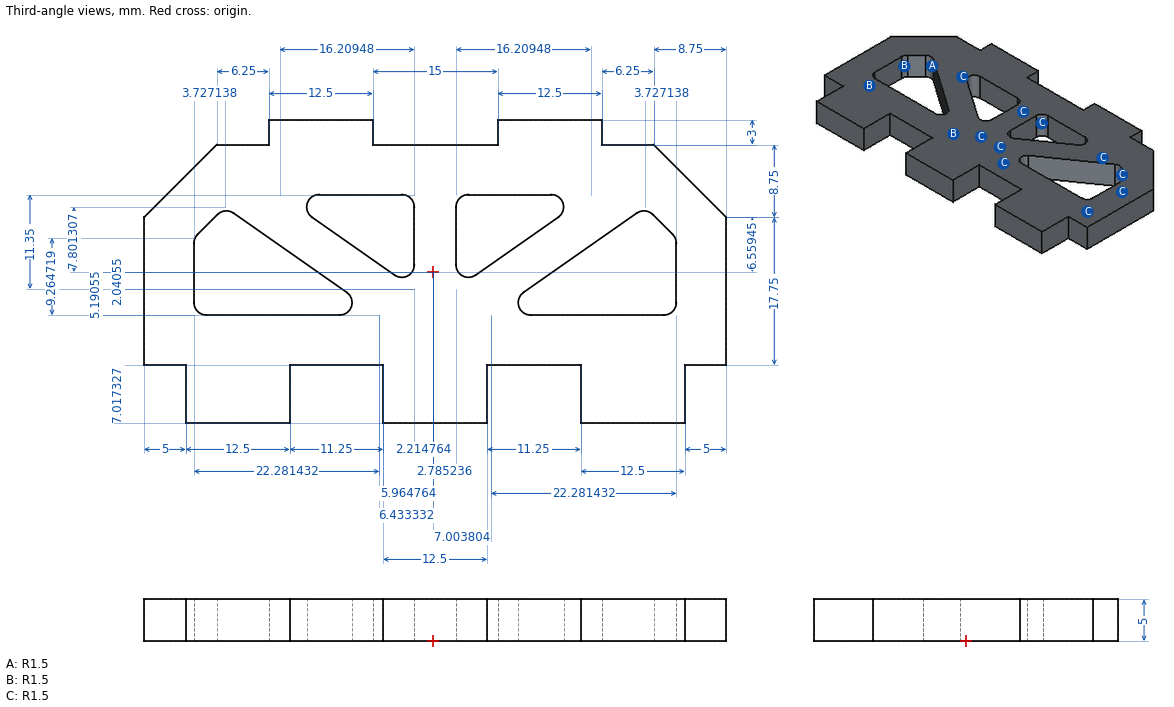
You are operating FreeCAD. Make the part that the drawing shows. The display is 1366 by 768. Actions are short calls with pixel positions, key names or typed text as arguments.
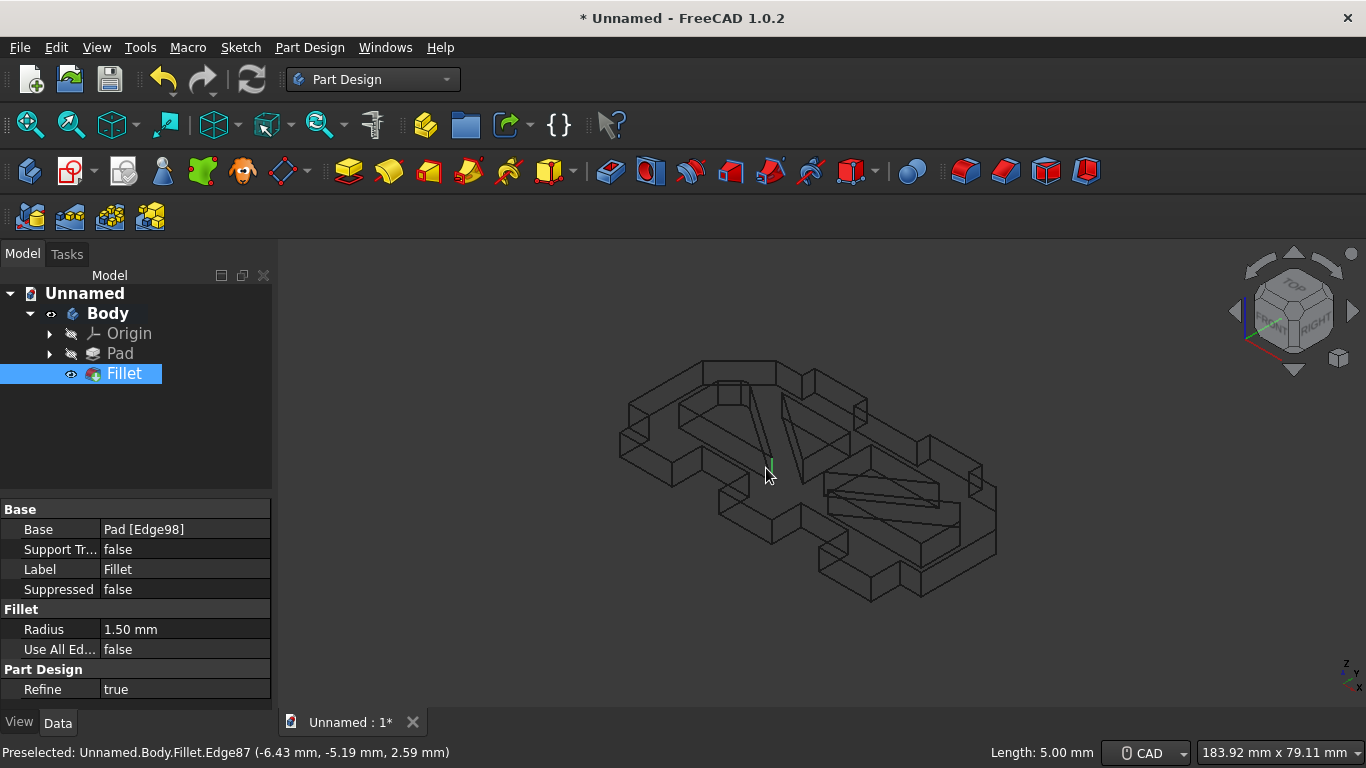
click(718, 392, ctrl)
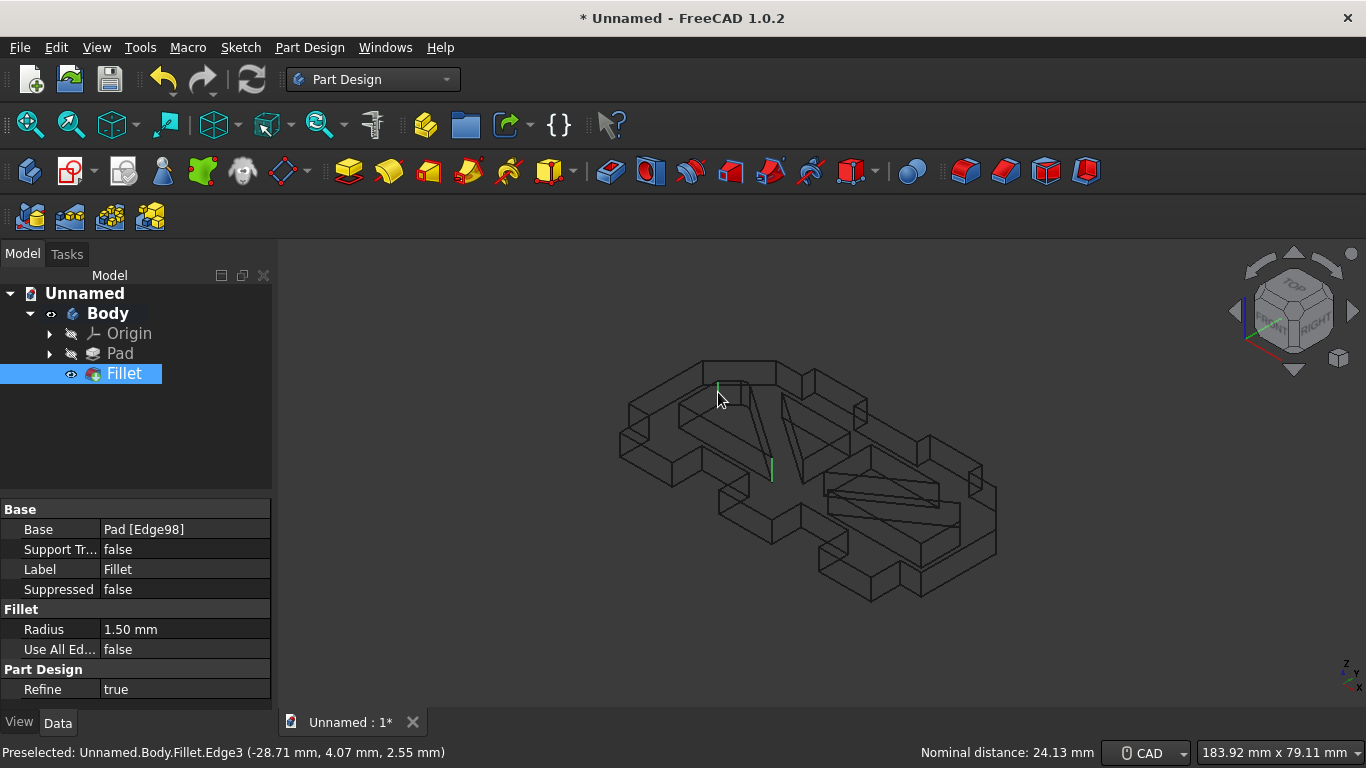
click(679, 415, ctrl)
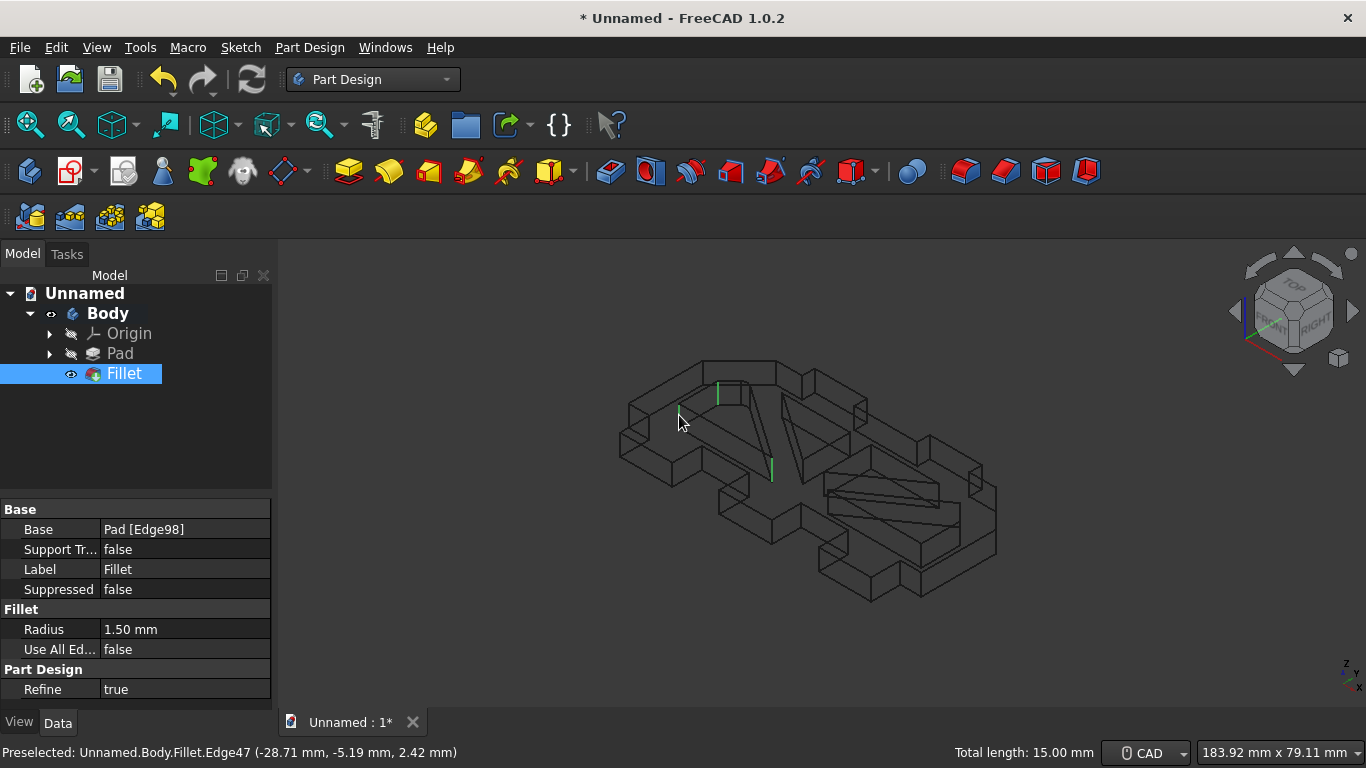
key(v)
key(1)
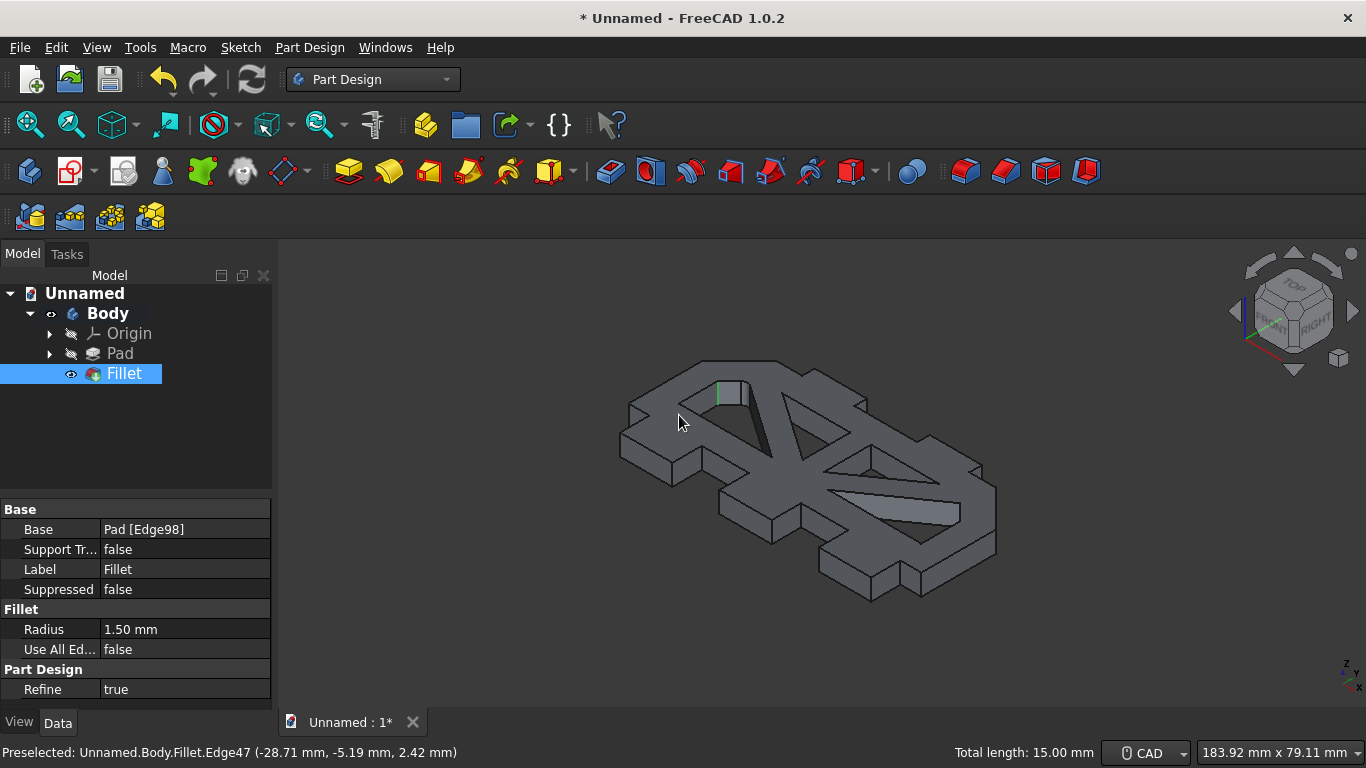
click(966, 172)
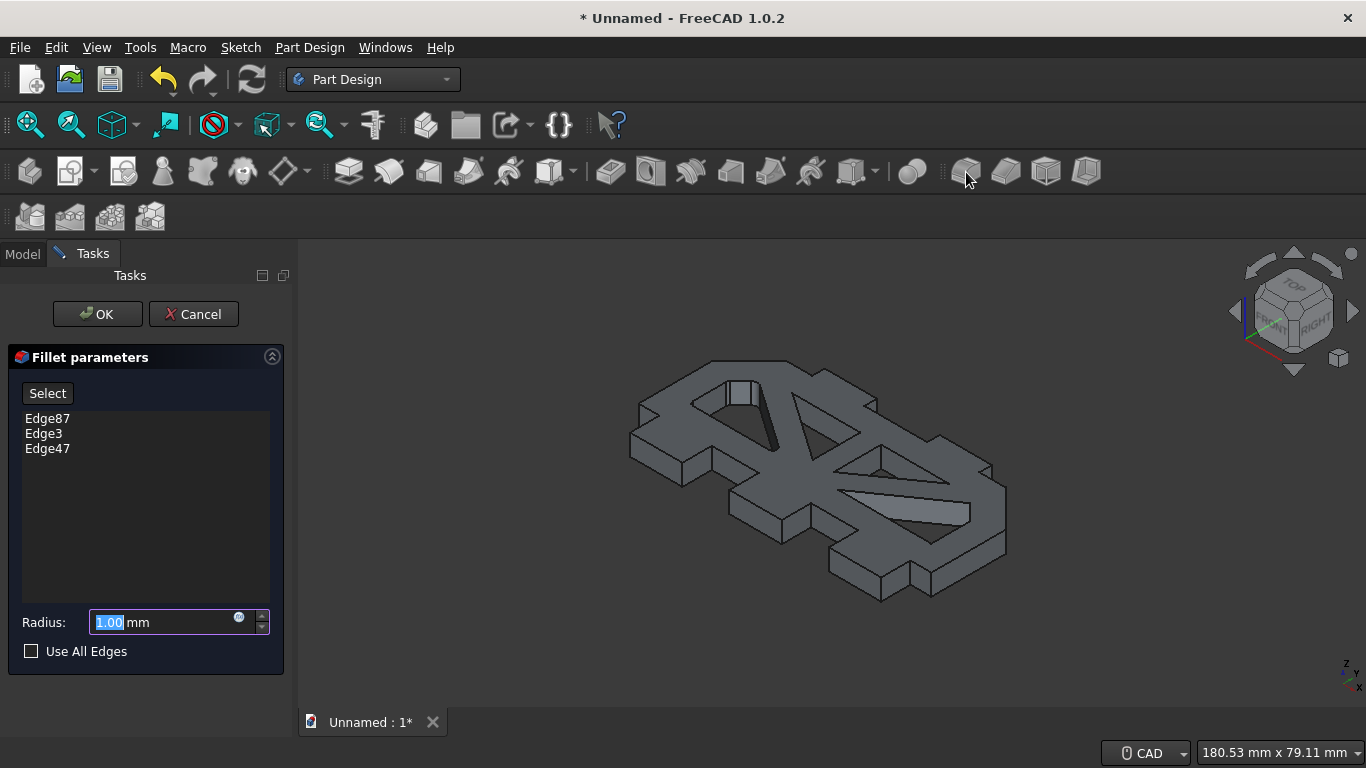
text(1.5)
key(Tab)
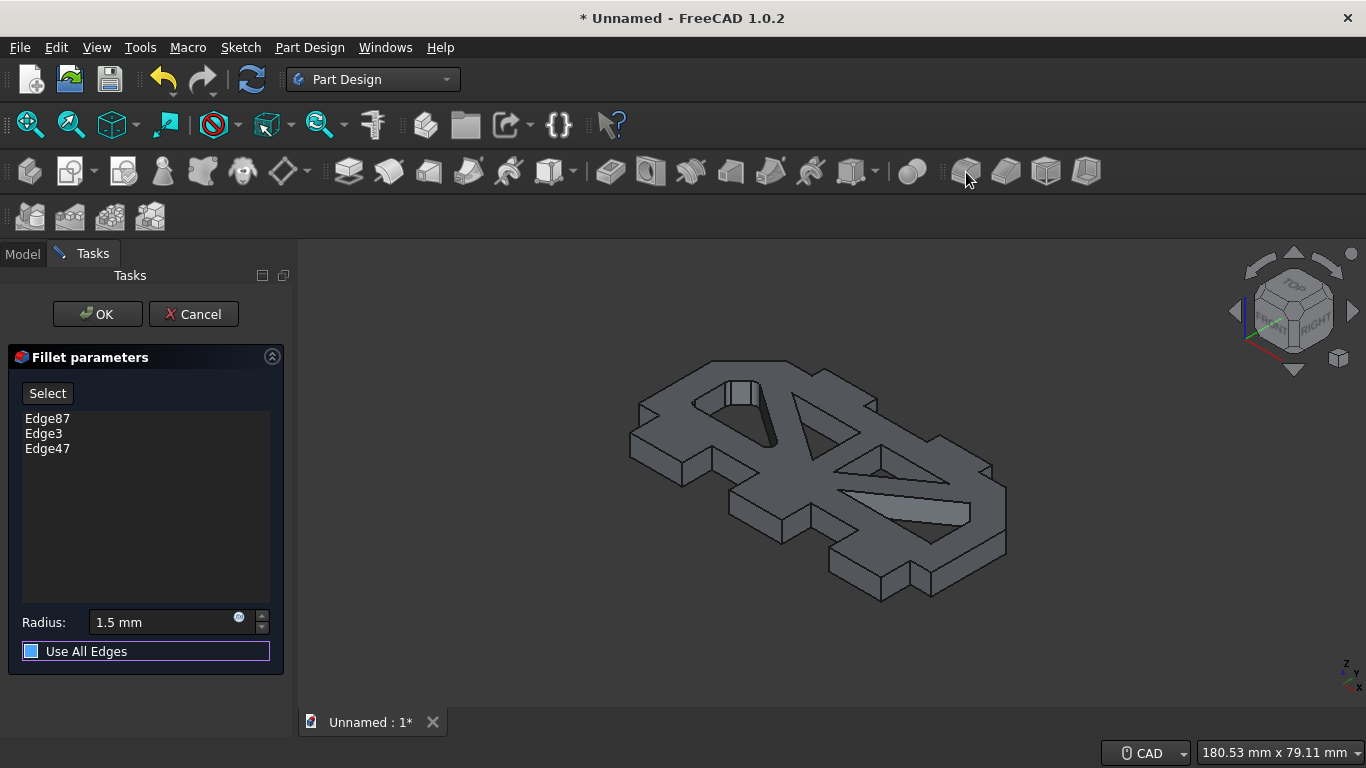
click(98, 314)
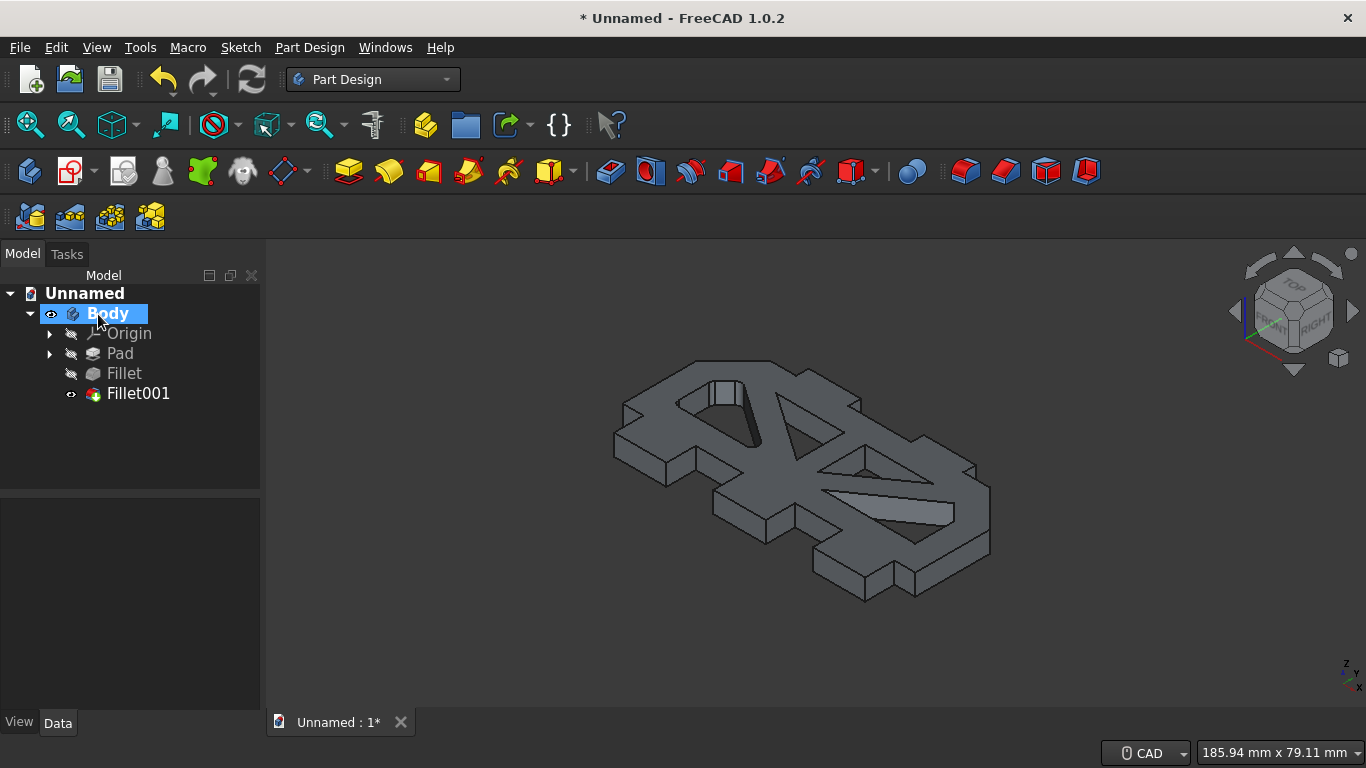
key(2)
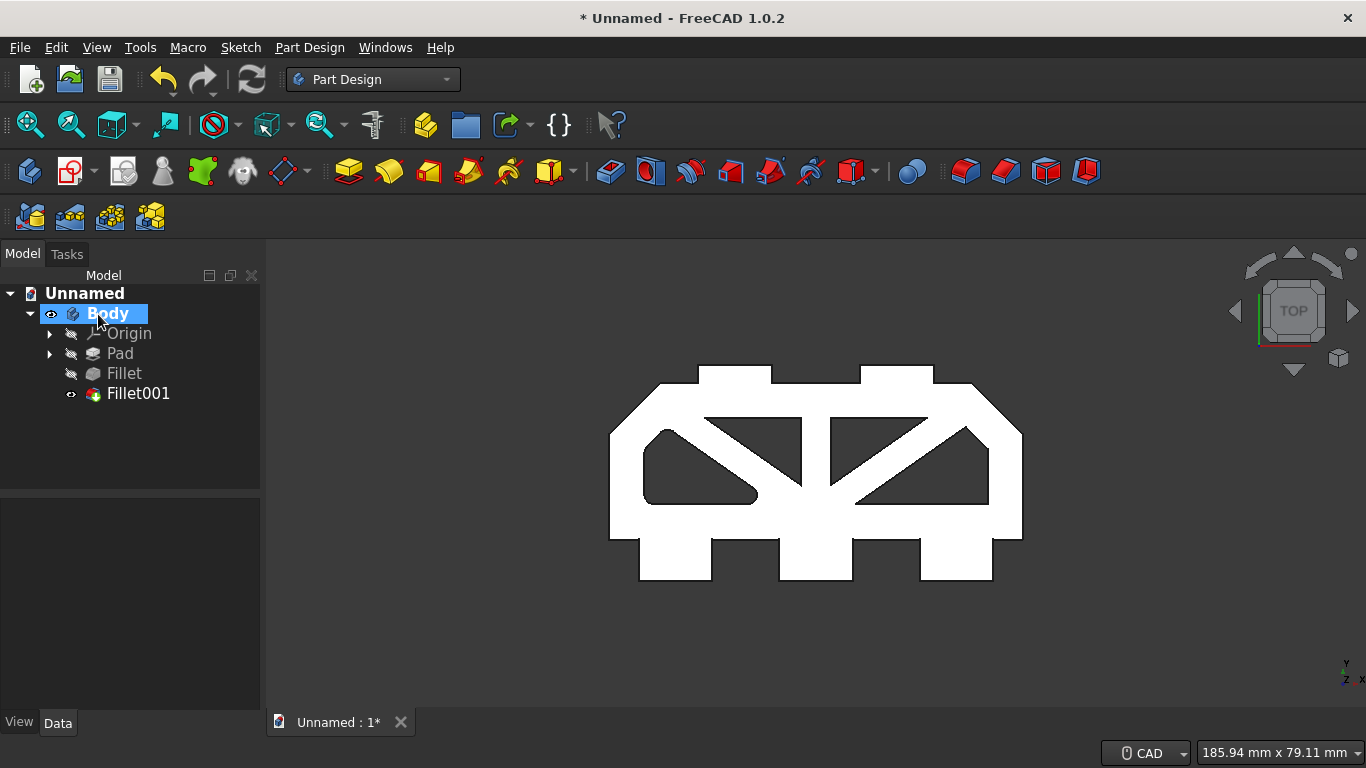
key(0)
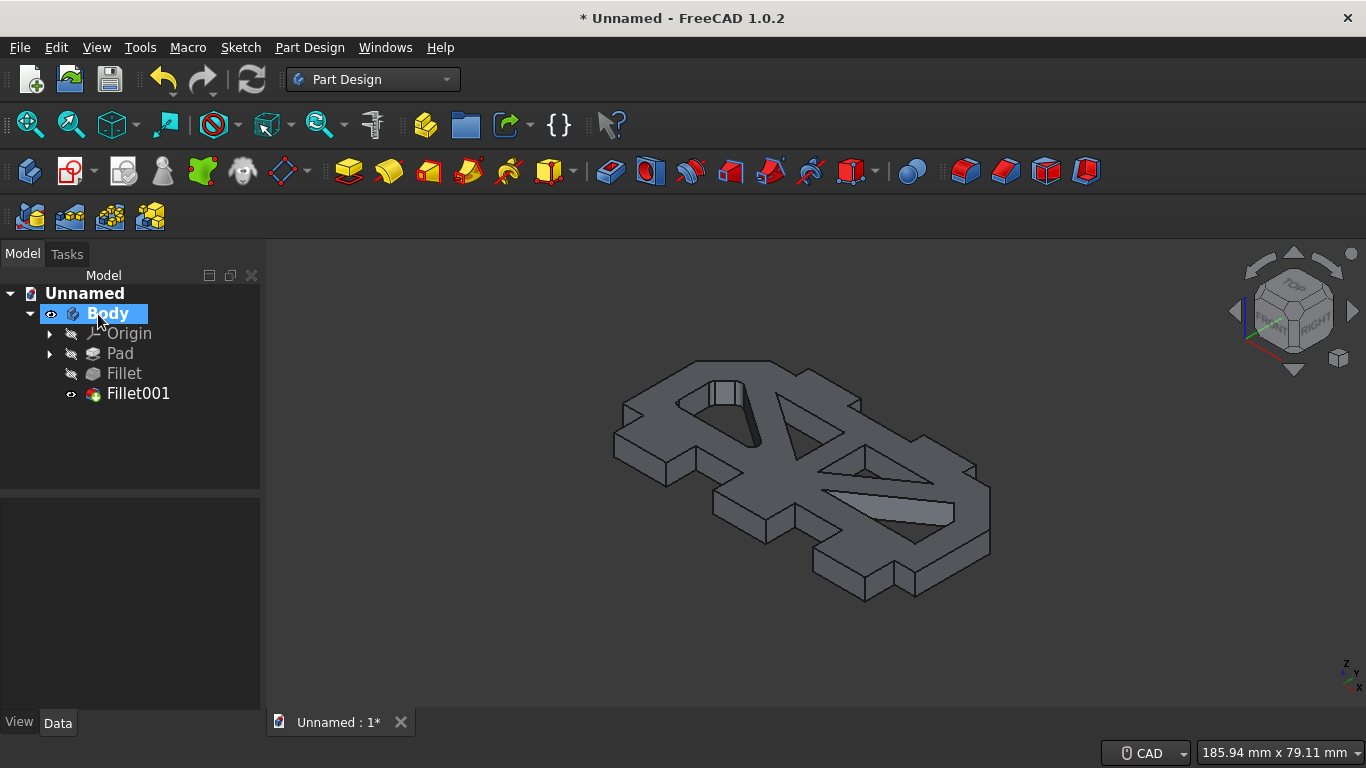
key(1)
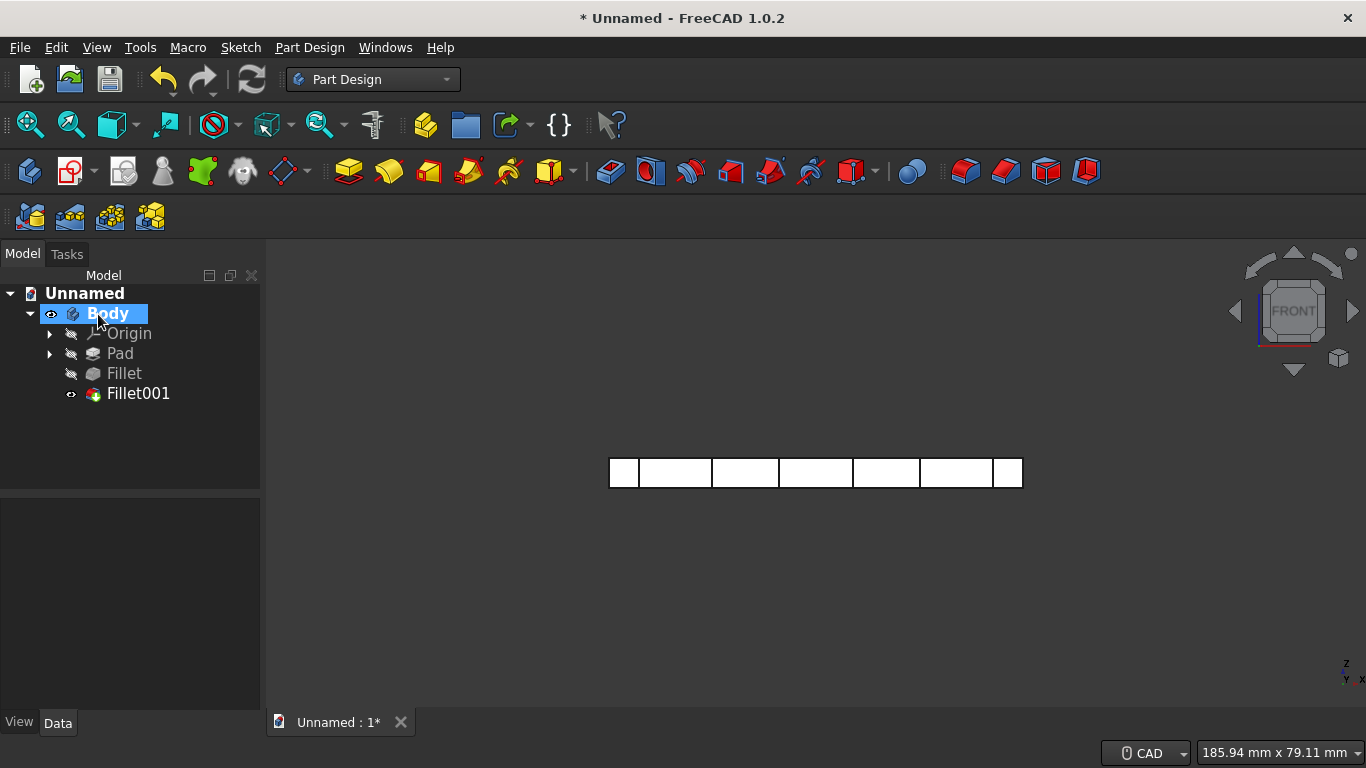
key(v)
key(f)